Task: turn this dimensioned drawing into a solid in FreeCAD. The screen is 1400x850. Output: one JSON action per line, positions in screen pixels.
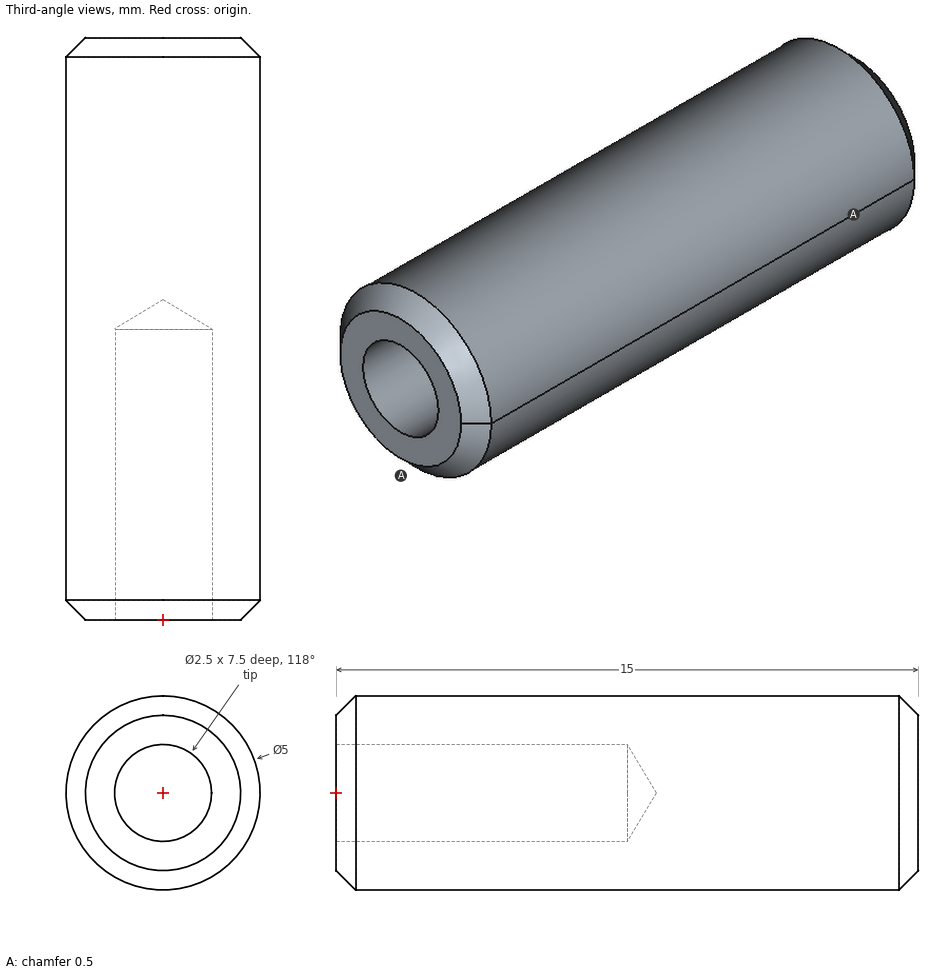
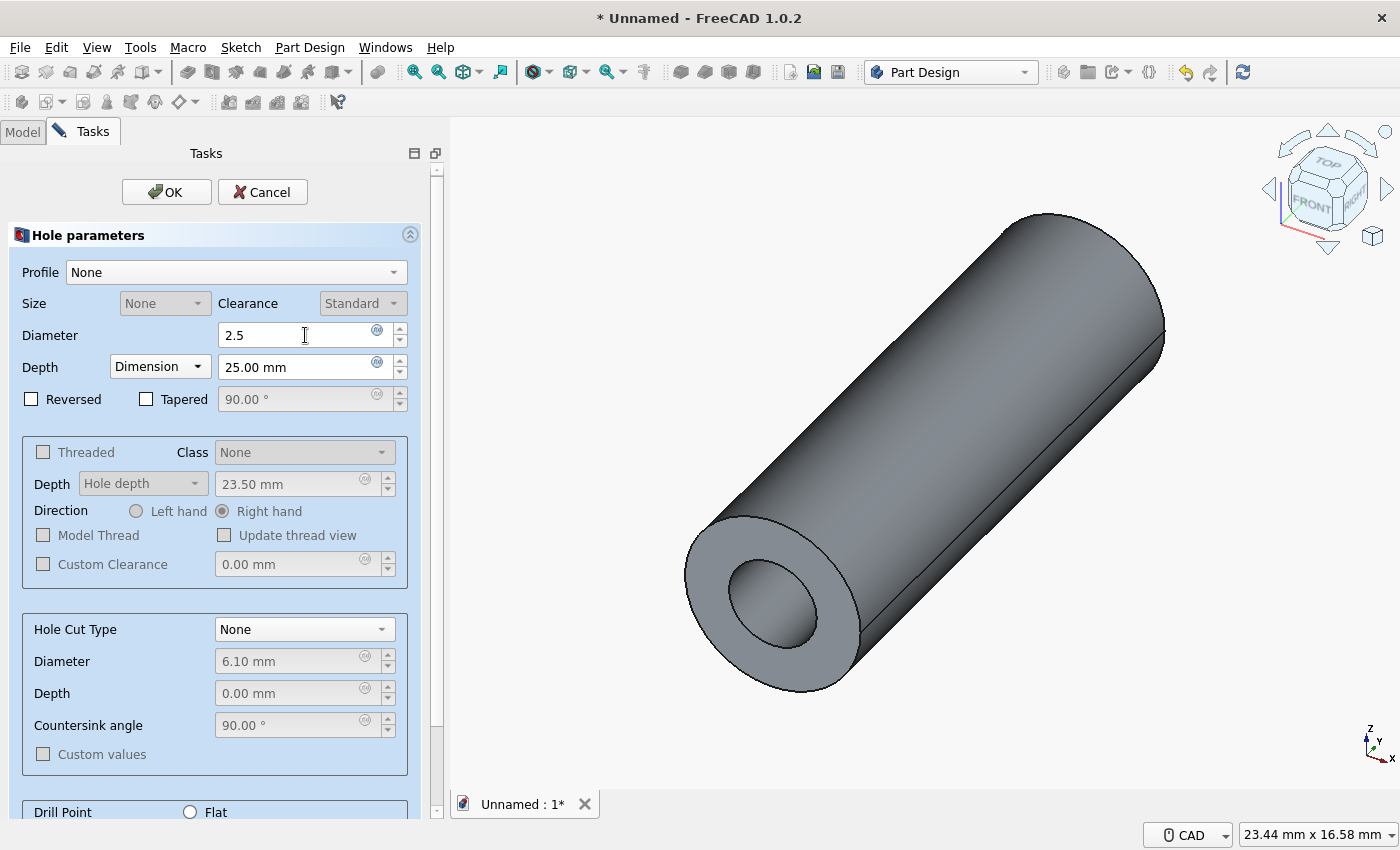
{"action": "triple_click", "coordinate": [305, 367]}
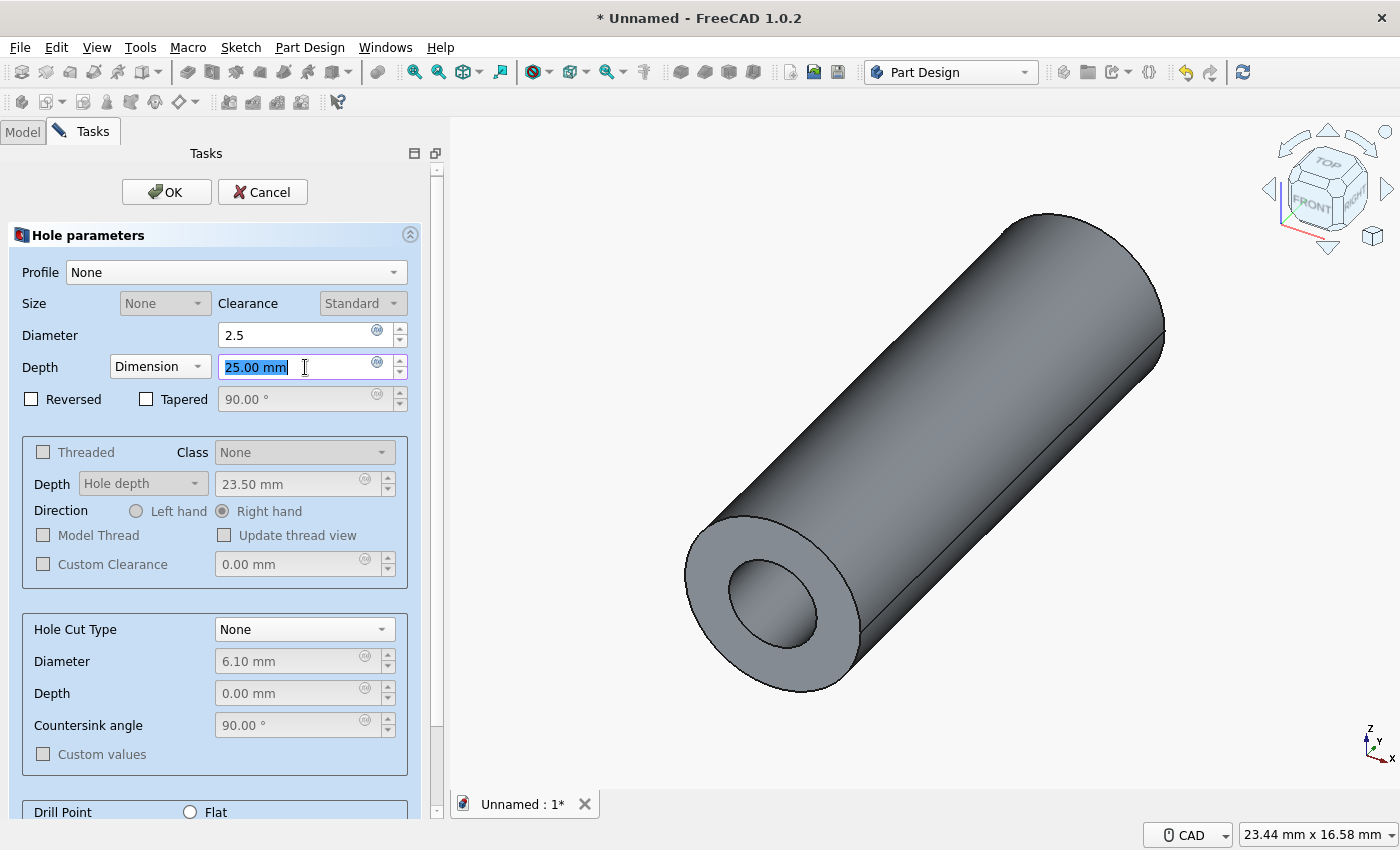
{"action": "type", "text": "7.5"}
{"action": "key", "text": "Tab"}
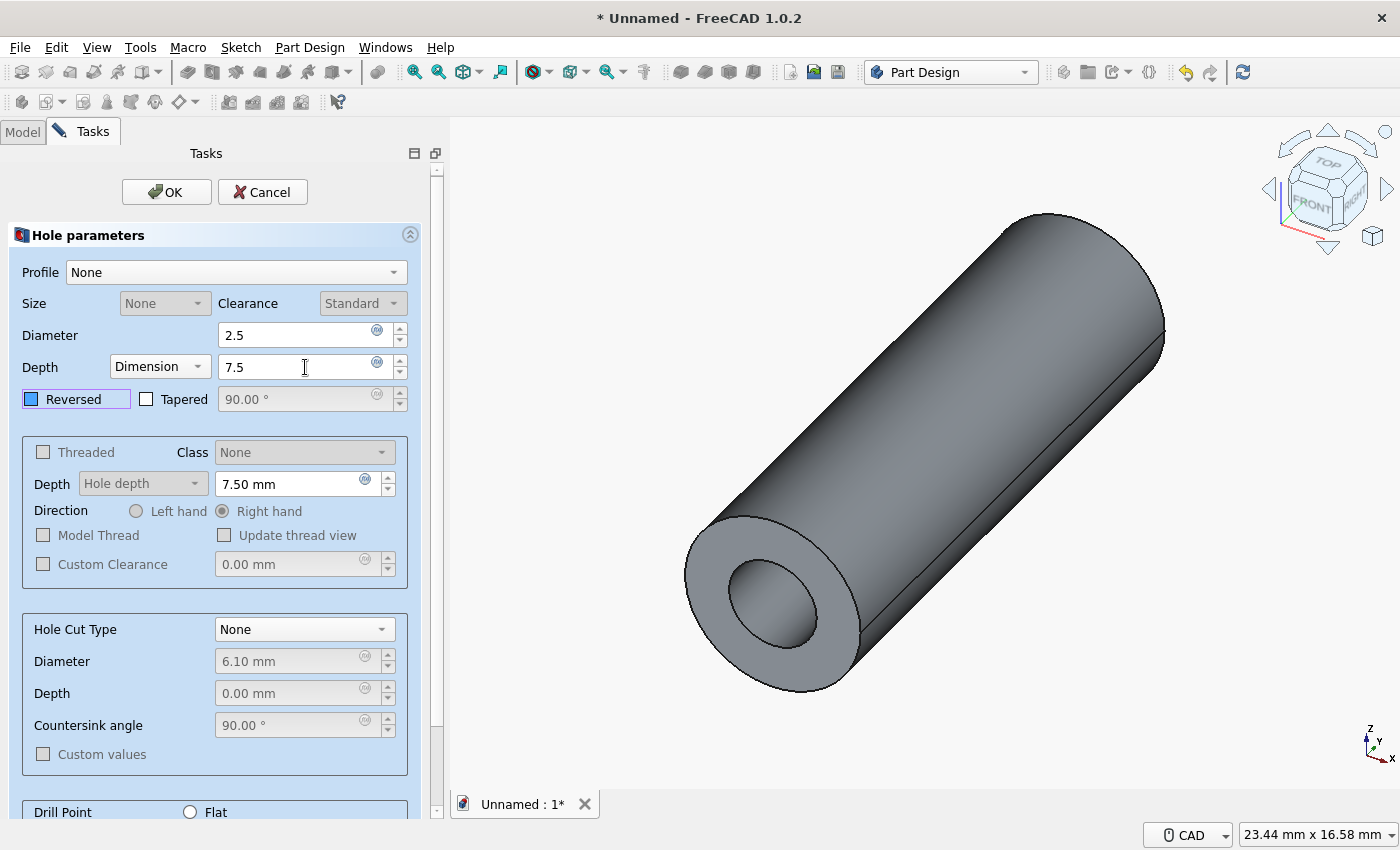
{"action": "left_click", "coordinate": [167, 192]}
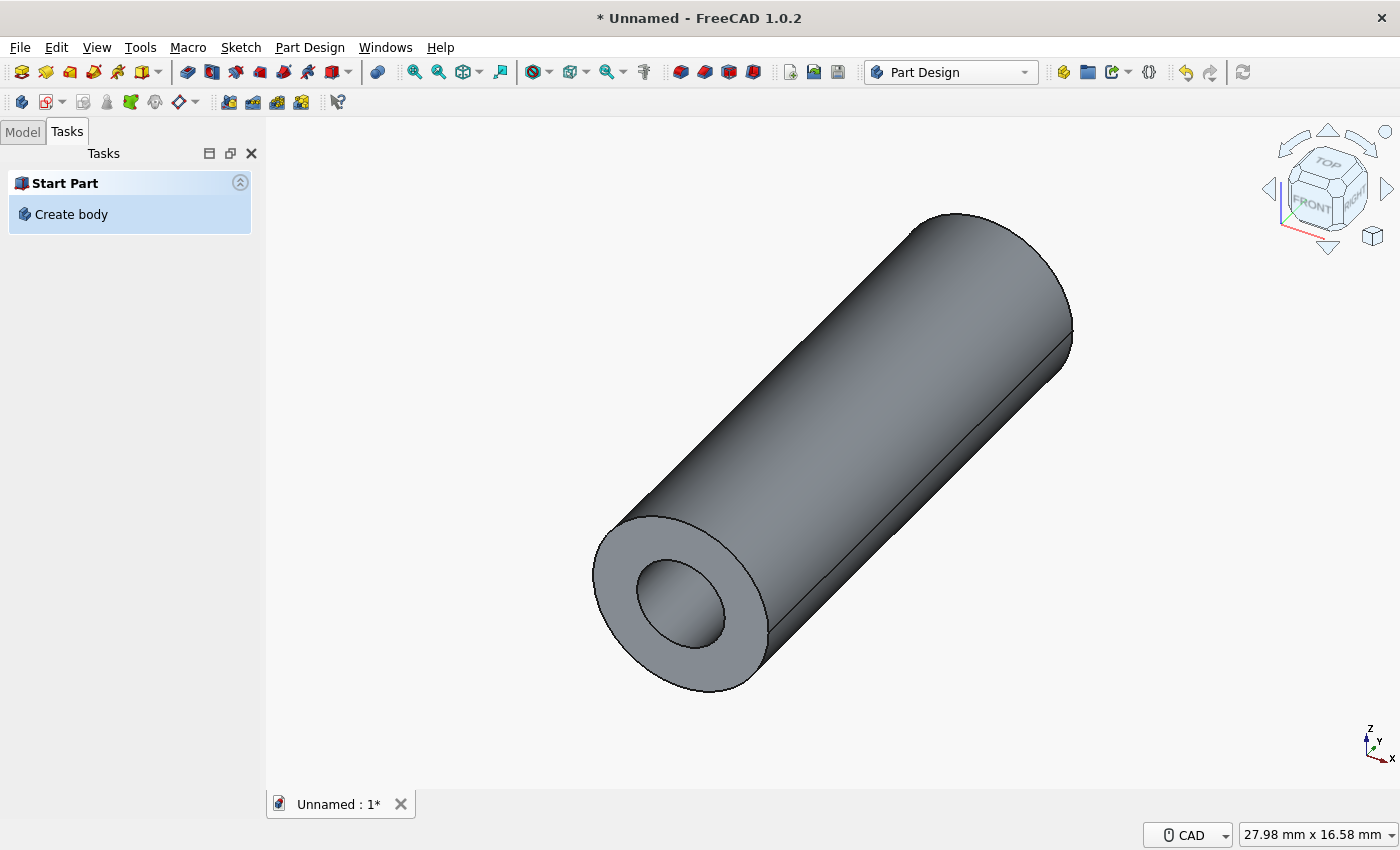
{"action": "left_click", "coordinate": [610, 531]}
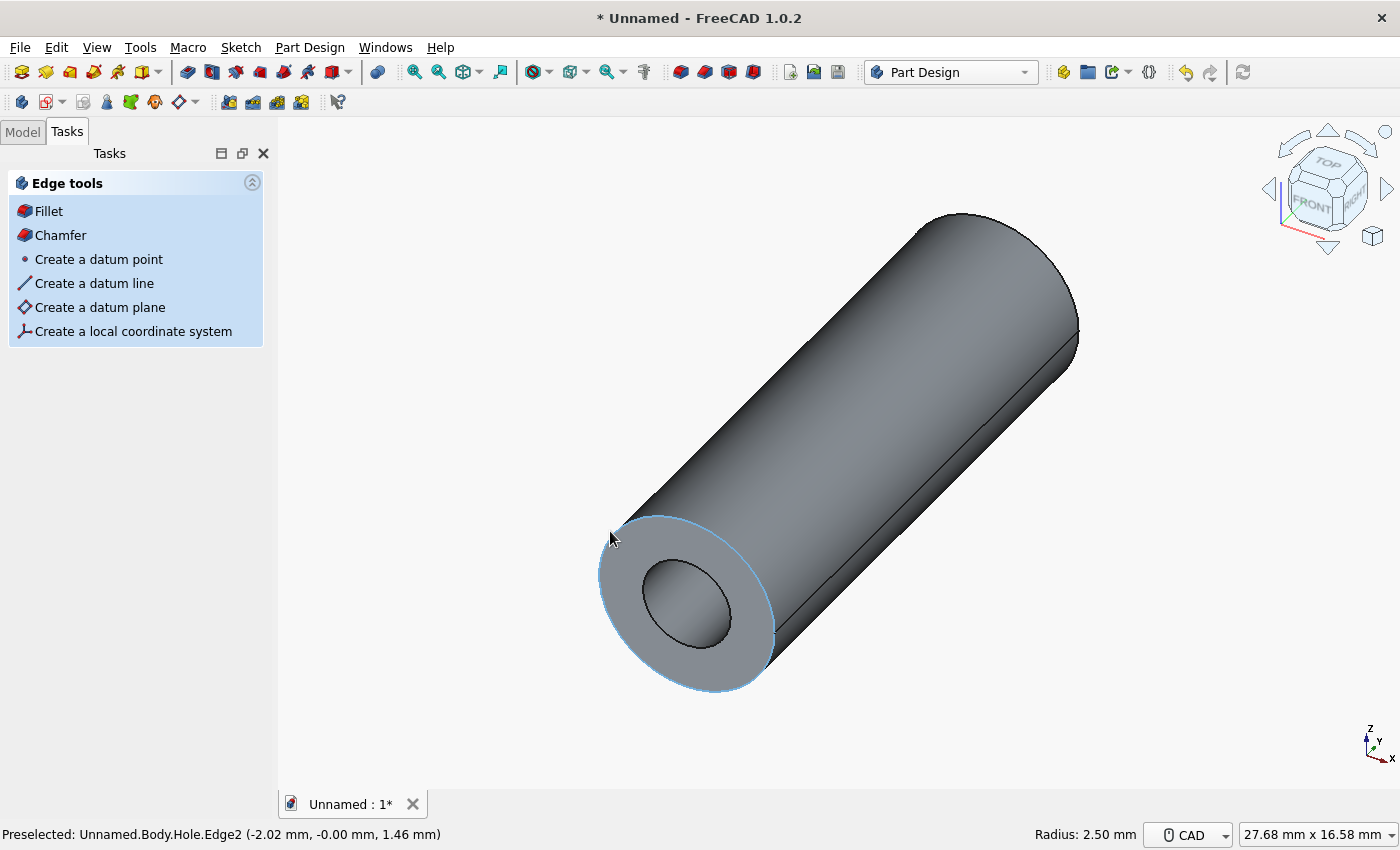
{"action": "key", "text": "0"}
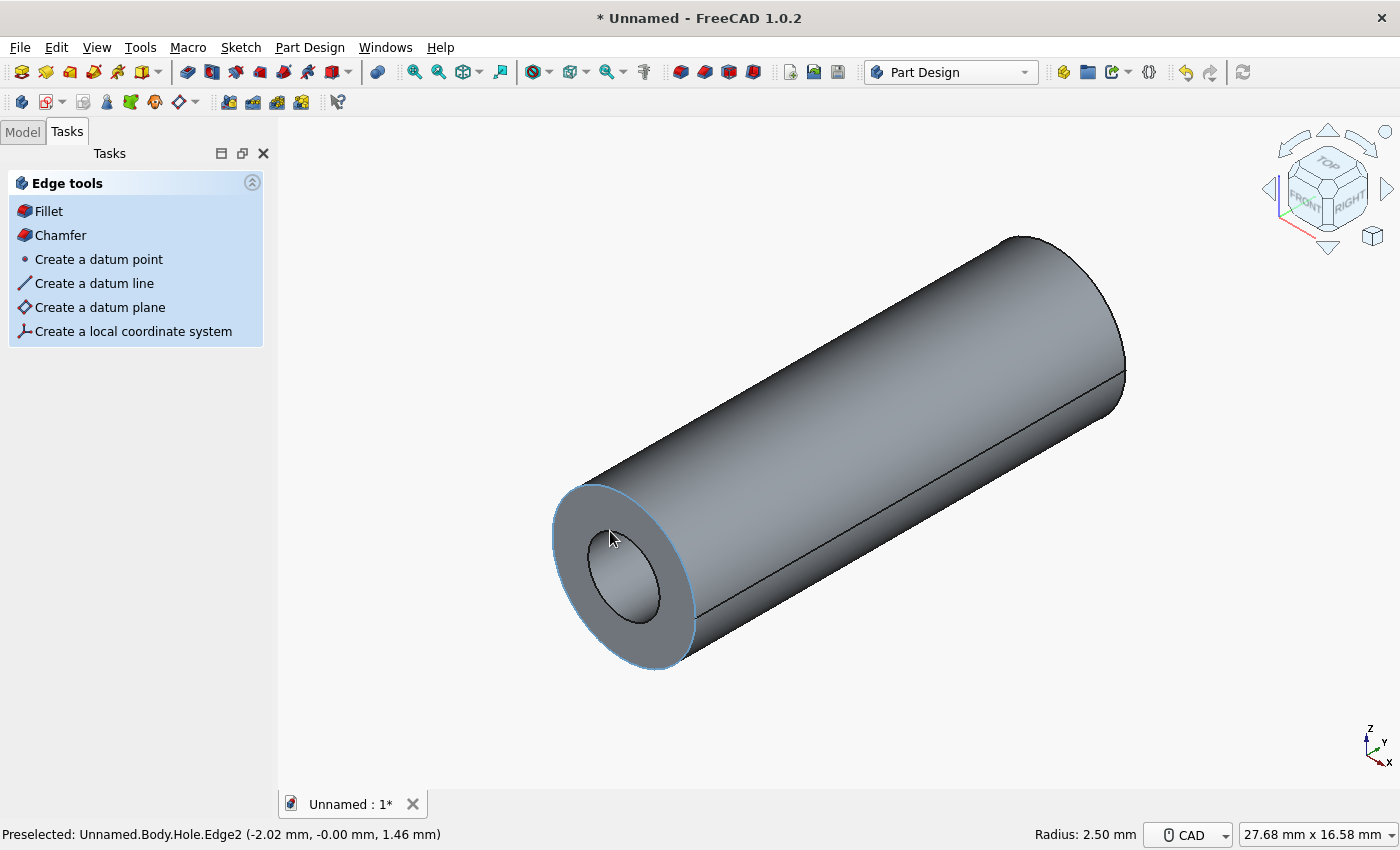
{"action": "key", "text": "2"}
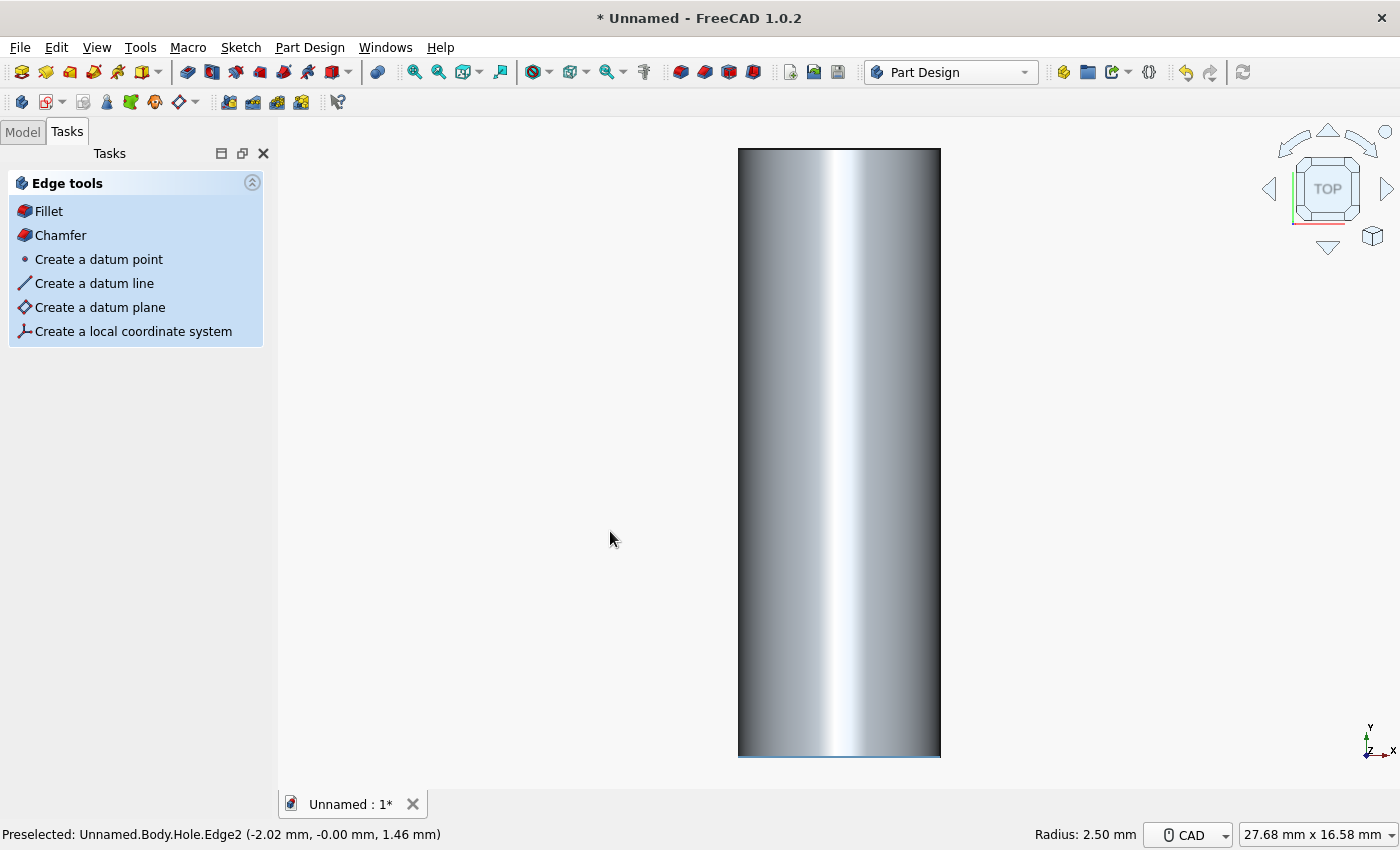
{"action": "left_click", "coordinate": [757, 148], "text": "ctrl"}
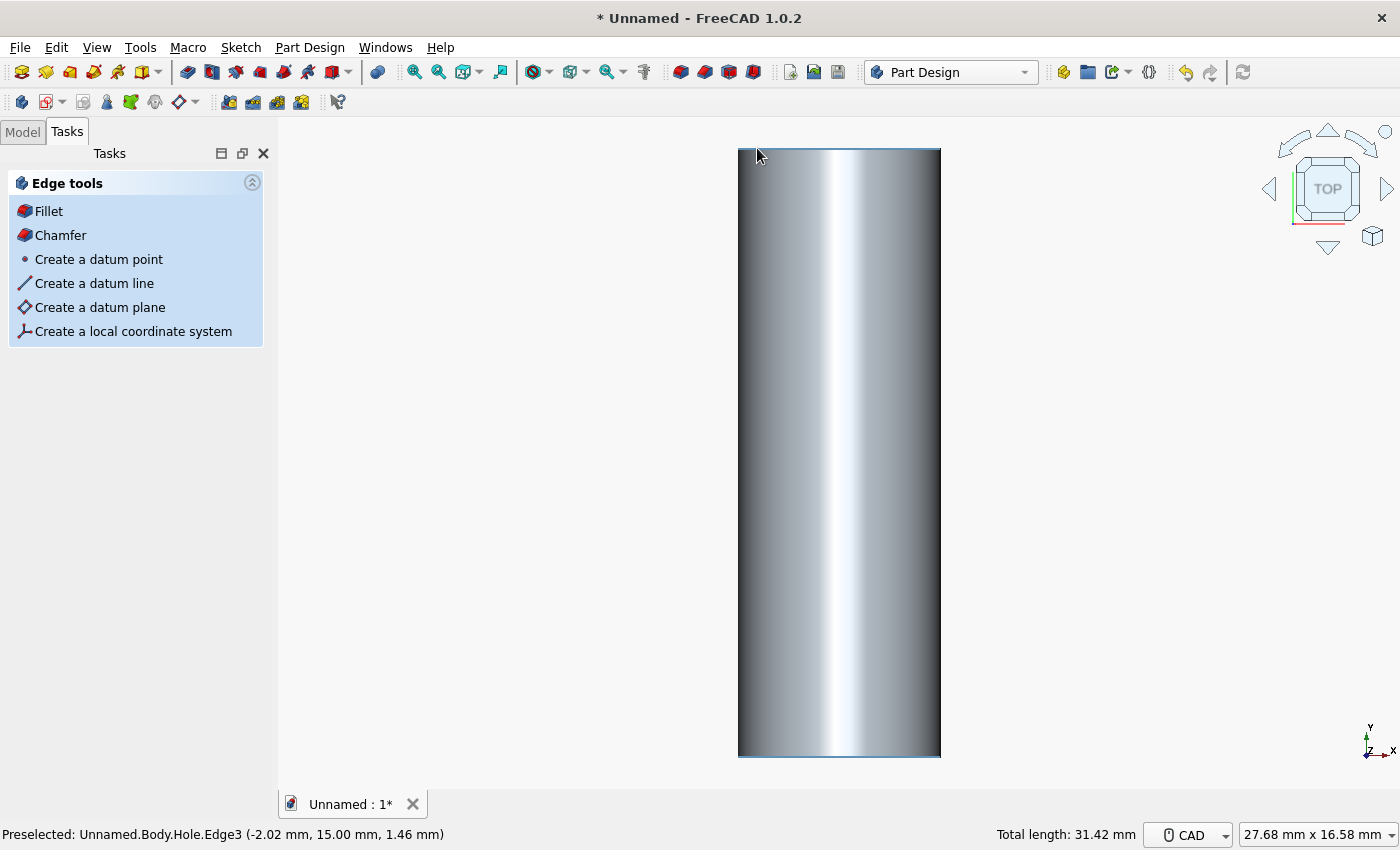
{"action": "left_click", "coordinate": [706, 72]}